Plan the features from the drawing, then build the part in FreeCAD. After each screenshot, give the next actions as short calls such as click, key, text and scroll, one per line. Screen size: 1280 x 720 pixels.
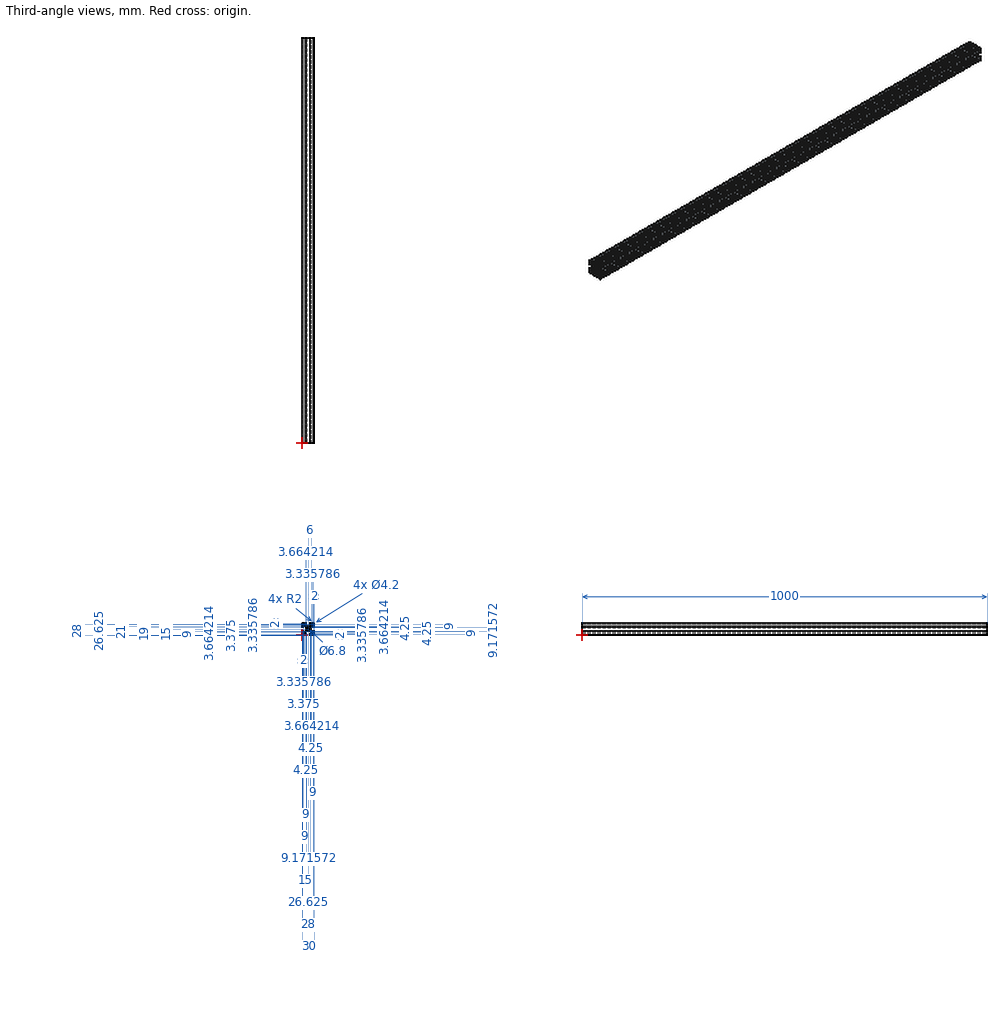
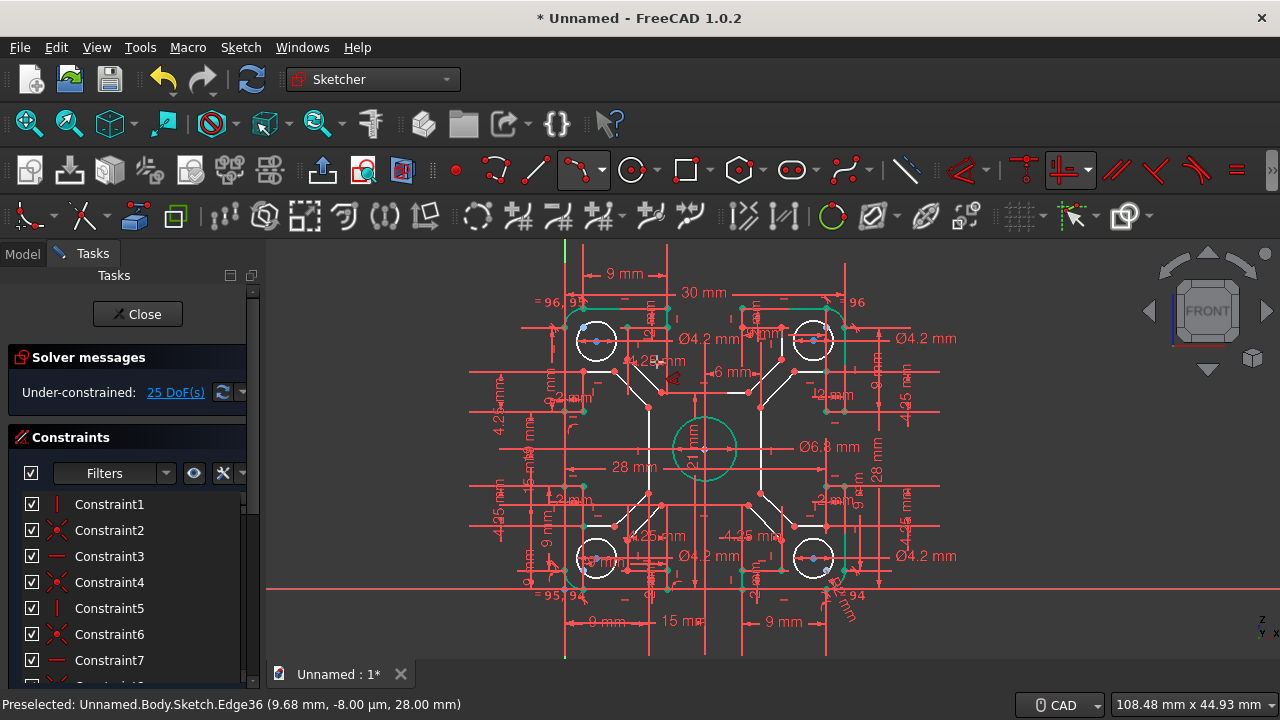
click(770, 328)
click(776, 294)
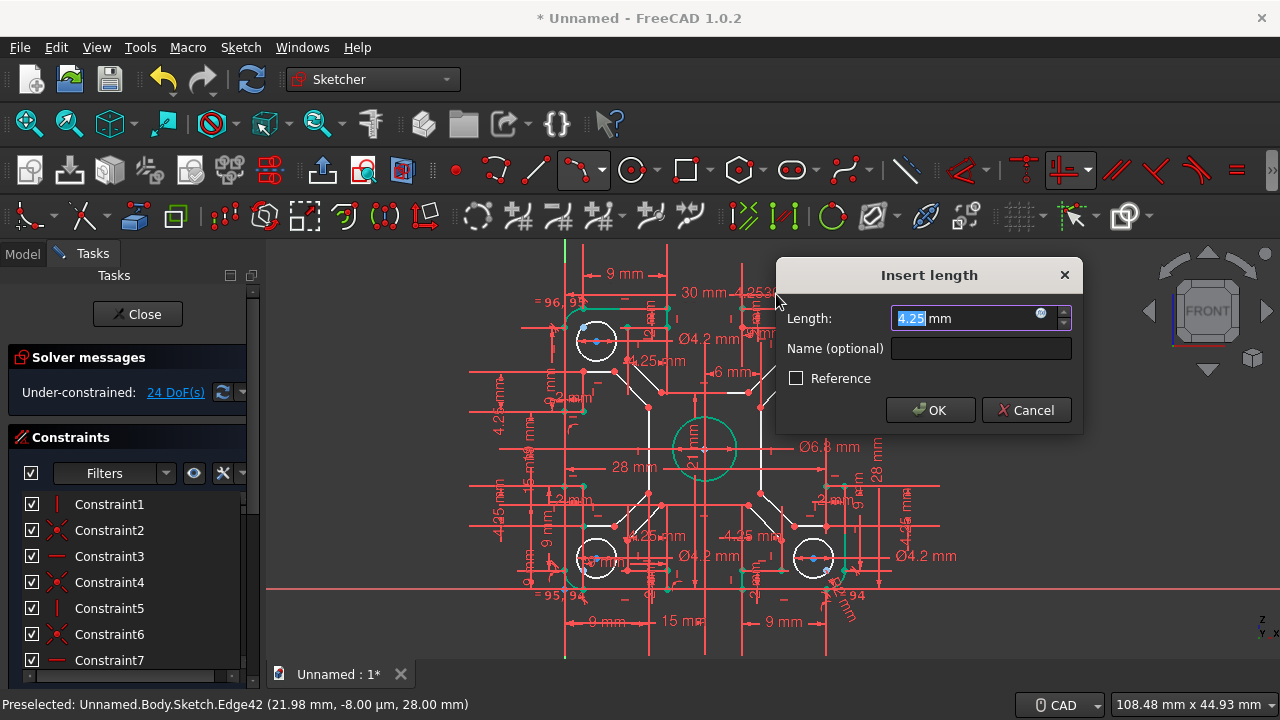
text(4.25)
key(Return)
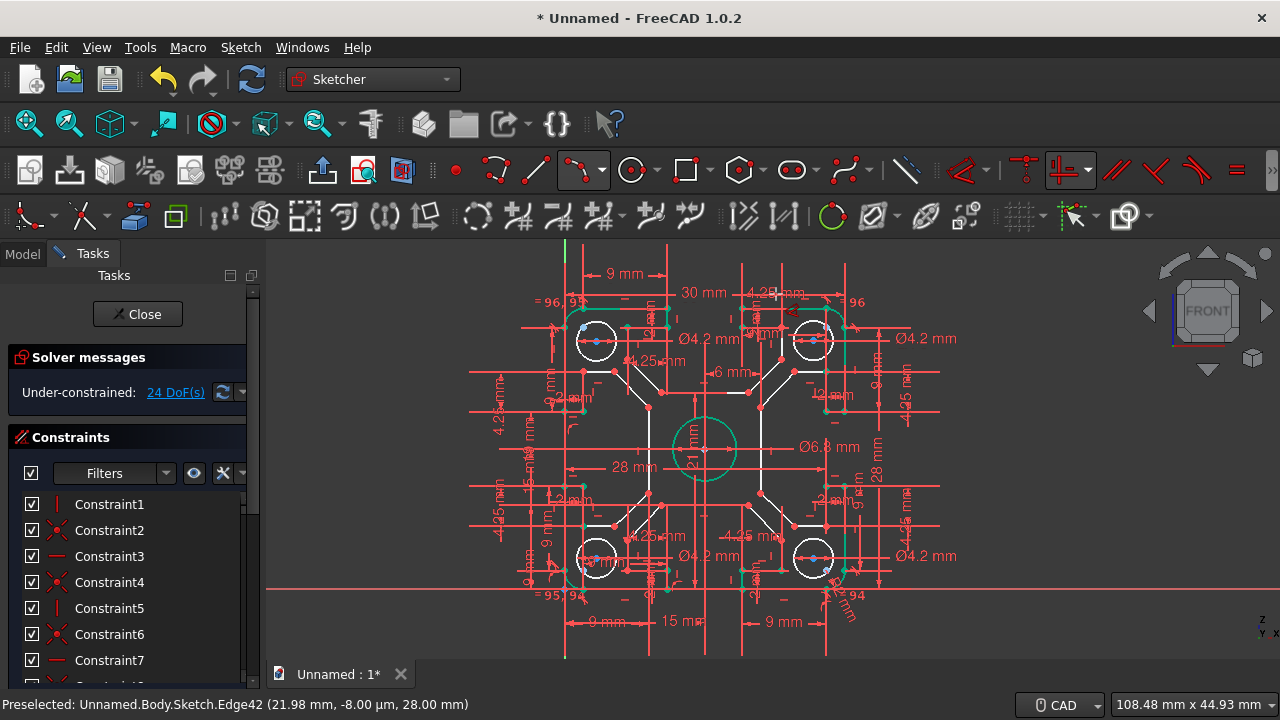
scroll(597, 341, up, 2)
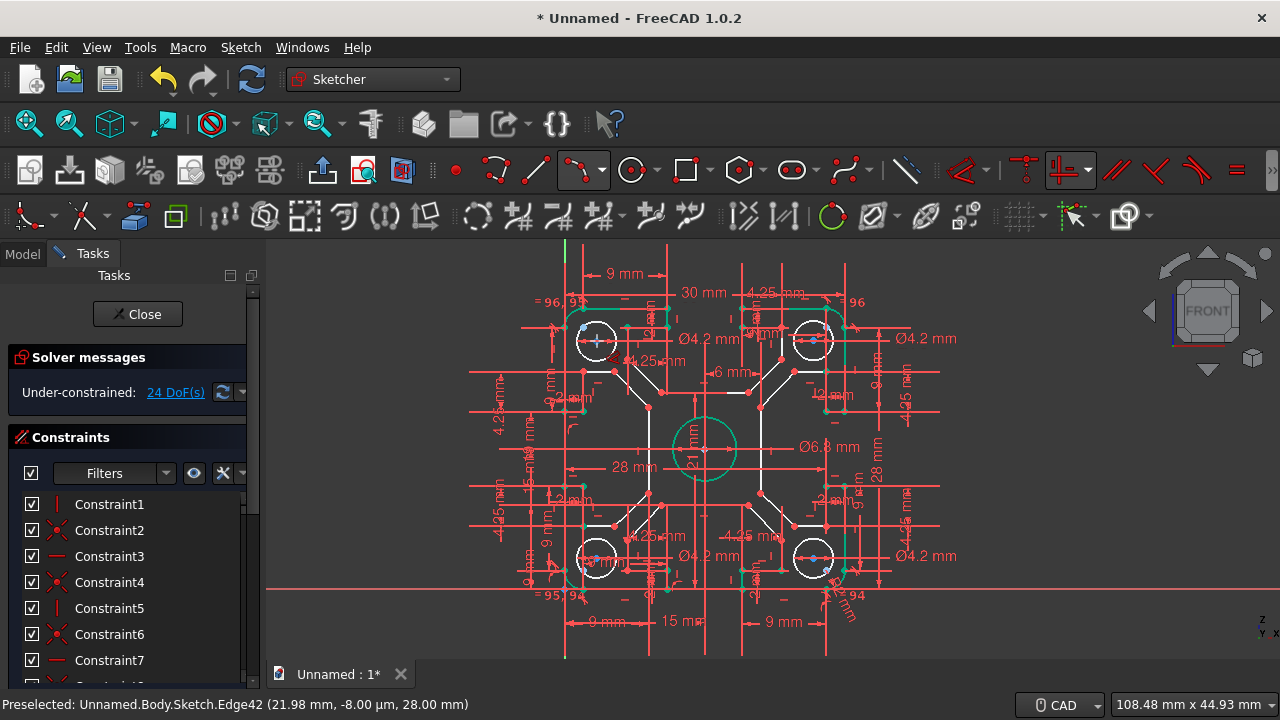
click(596, 341)
click(572, 307)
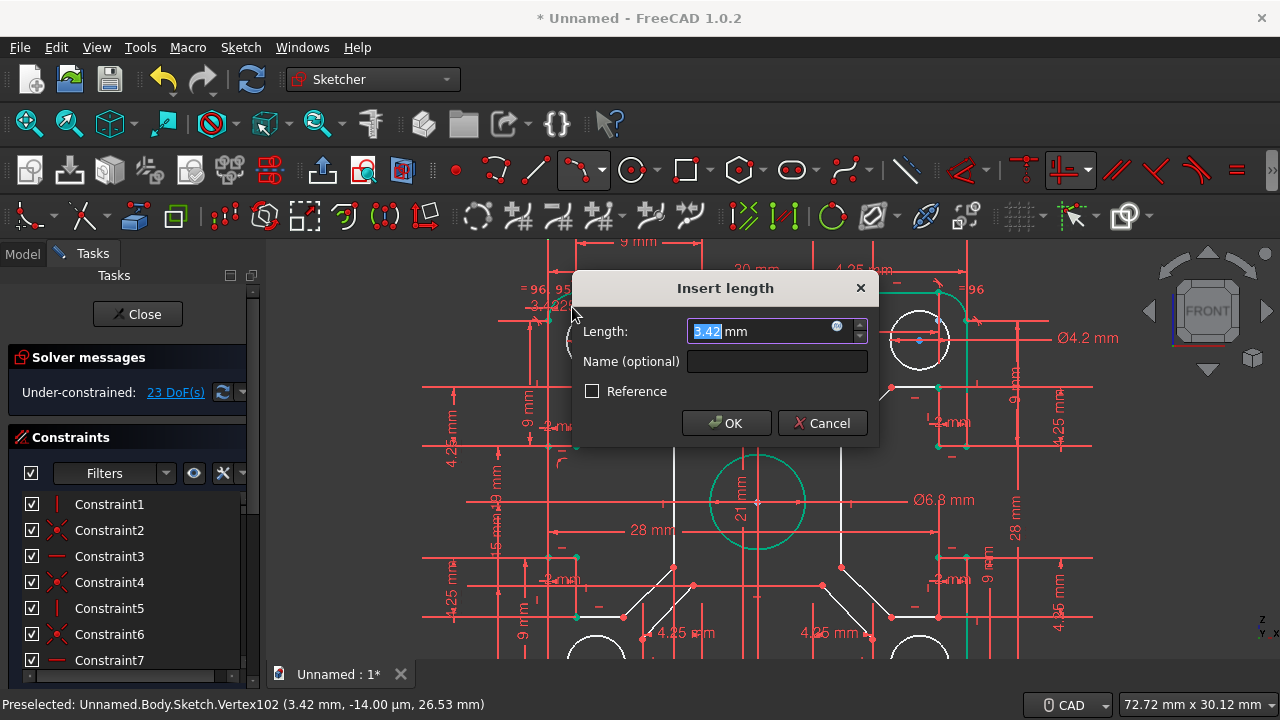
text(3.375)
key(Return)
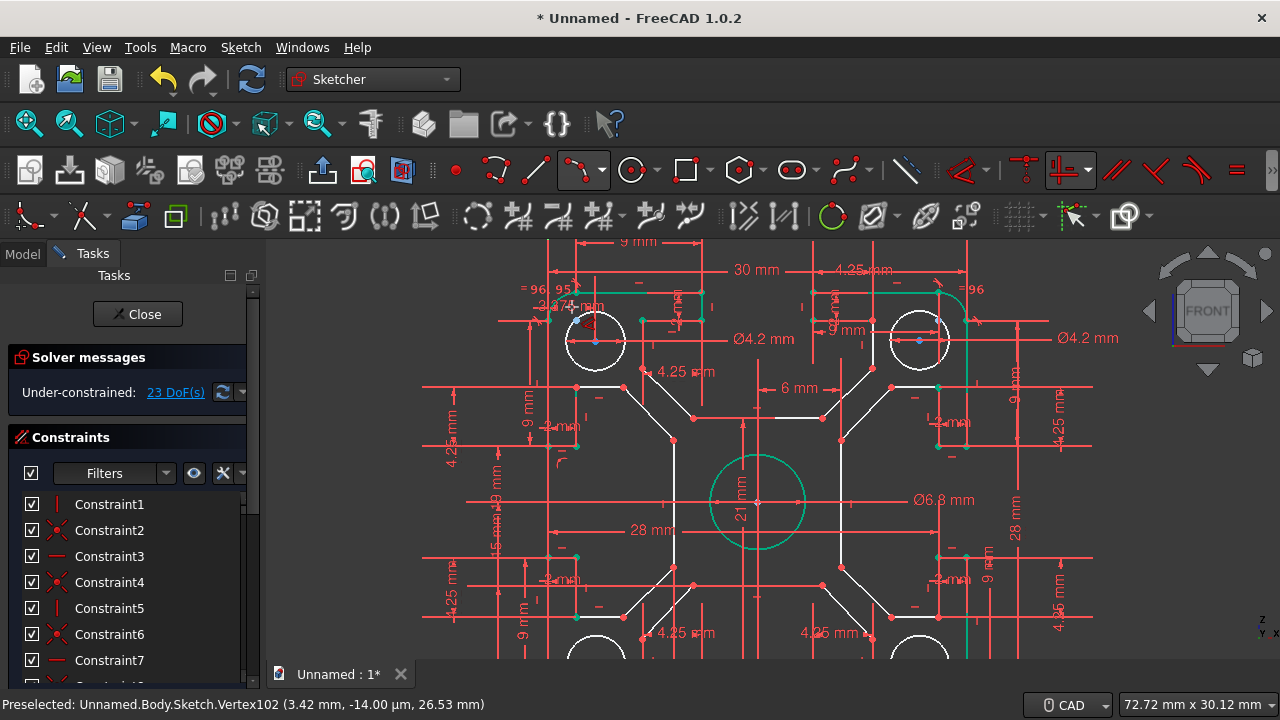
scroll(597, 341, down, 2)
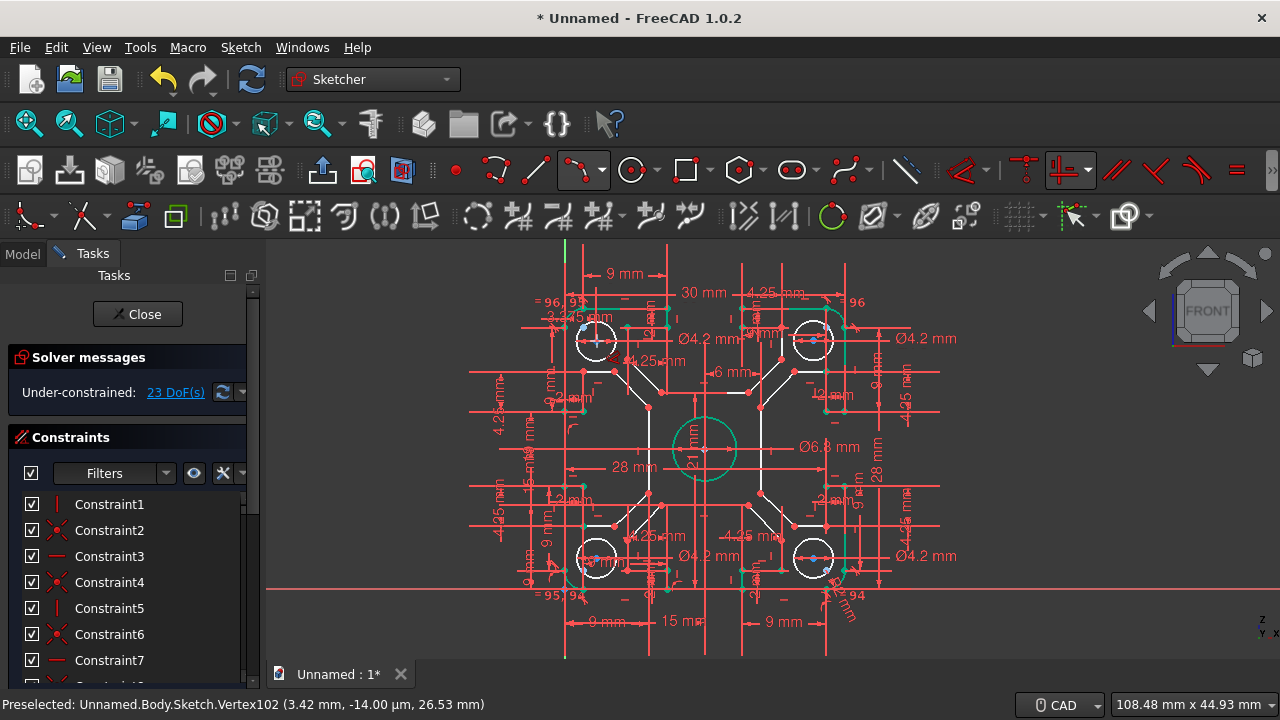
scroll(814, 558, up, 2)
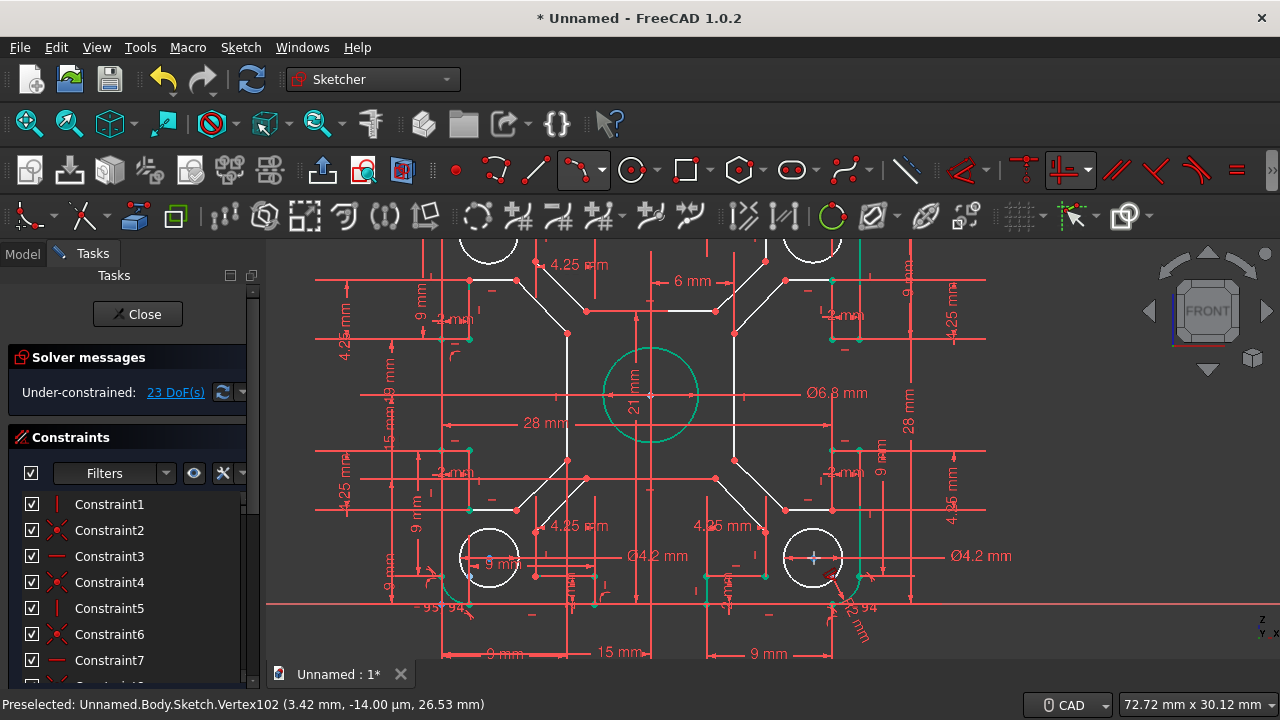
click(813, 558)
click(895, 581)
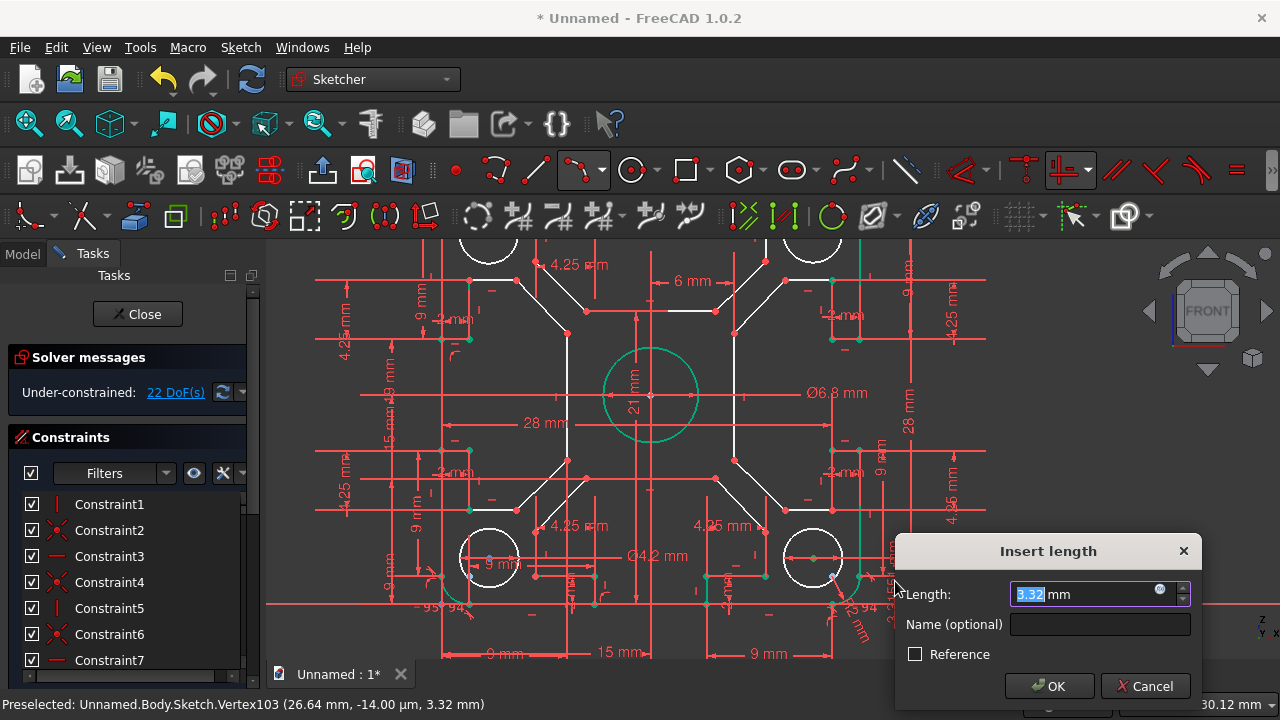
text(3.375)
key(Return)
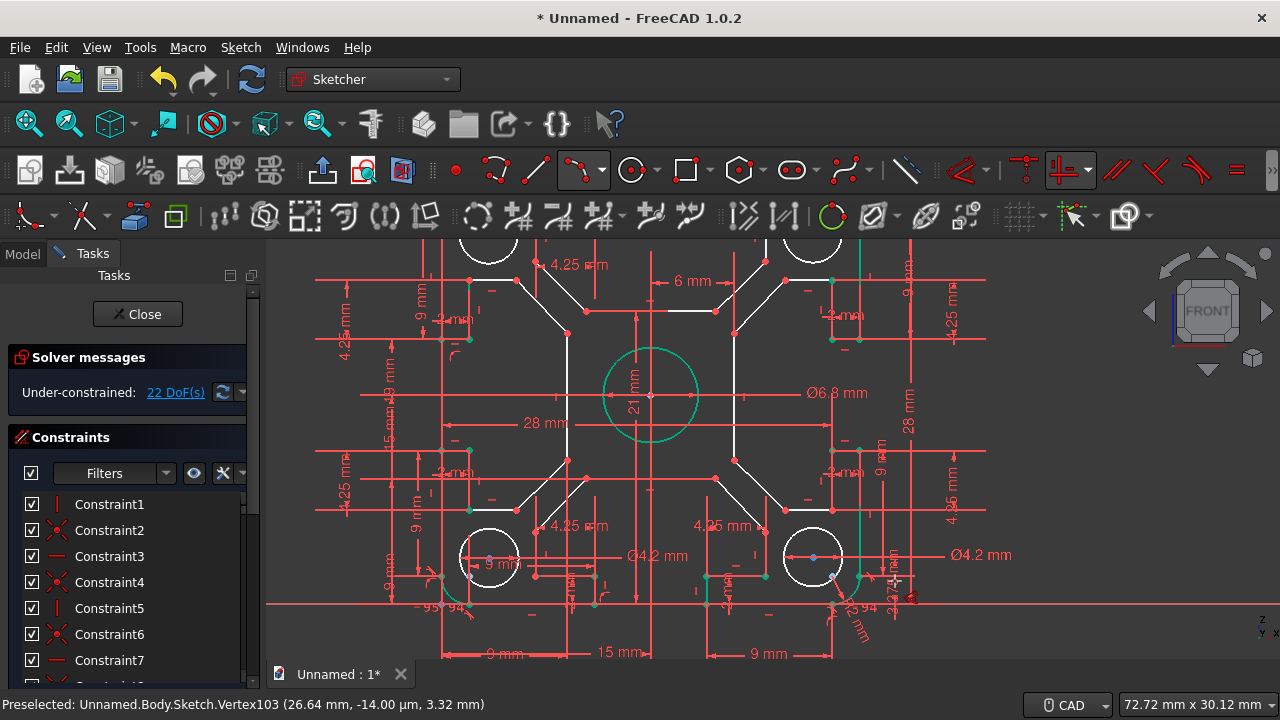
click(489, 558)
click(465, 428)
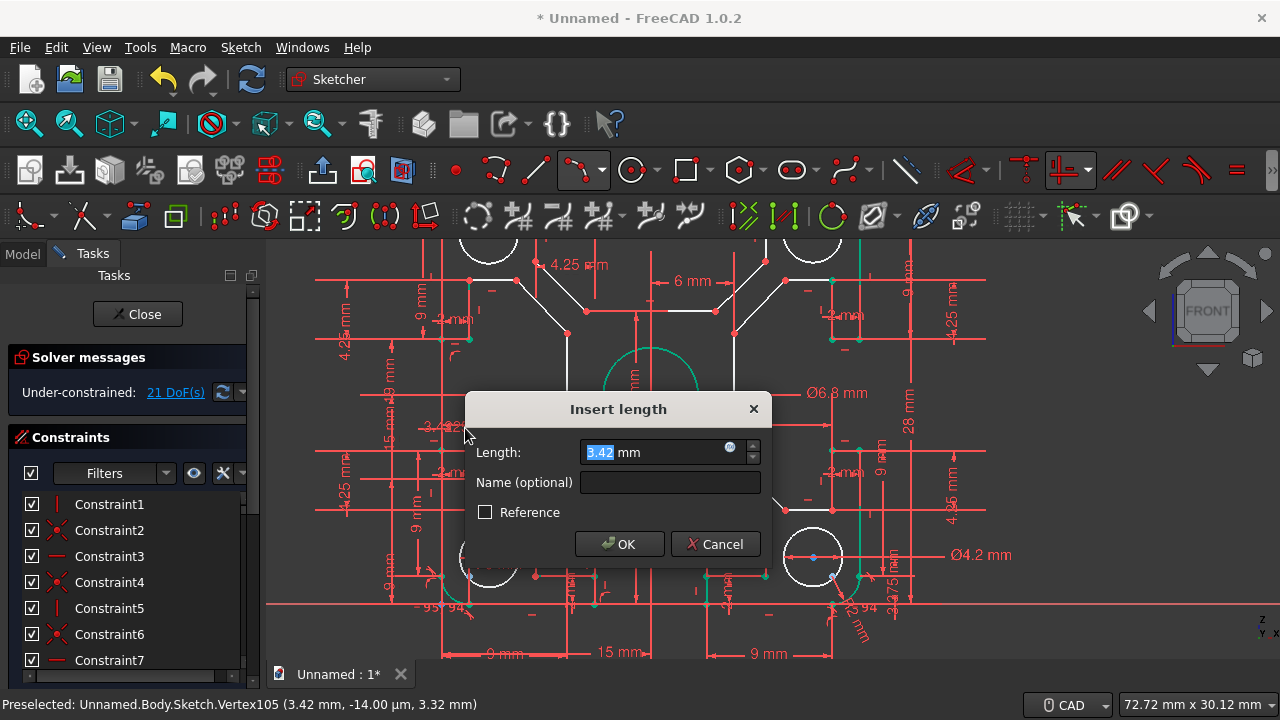
text(3.375)
key(Return)